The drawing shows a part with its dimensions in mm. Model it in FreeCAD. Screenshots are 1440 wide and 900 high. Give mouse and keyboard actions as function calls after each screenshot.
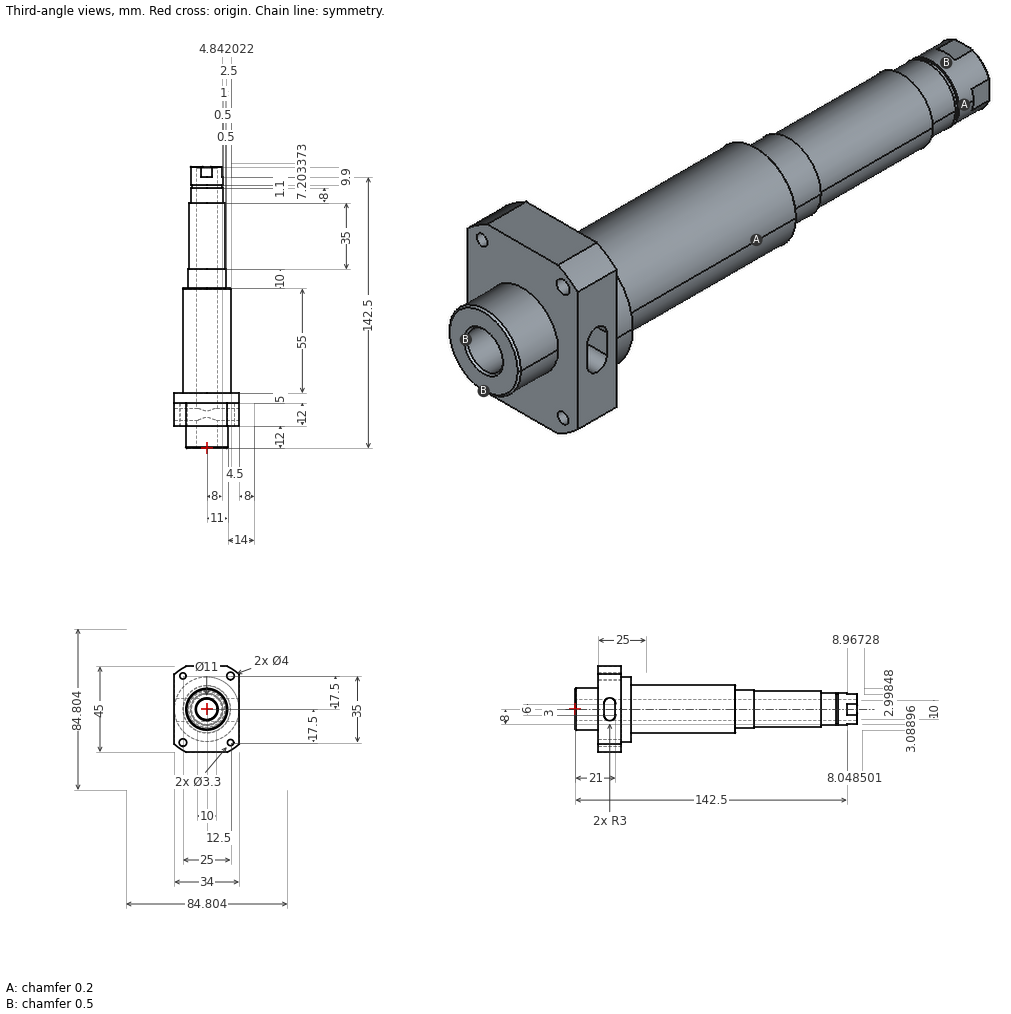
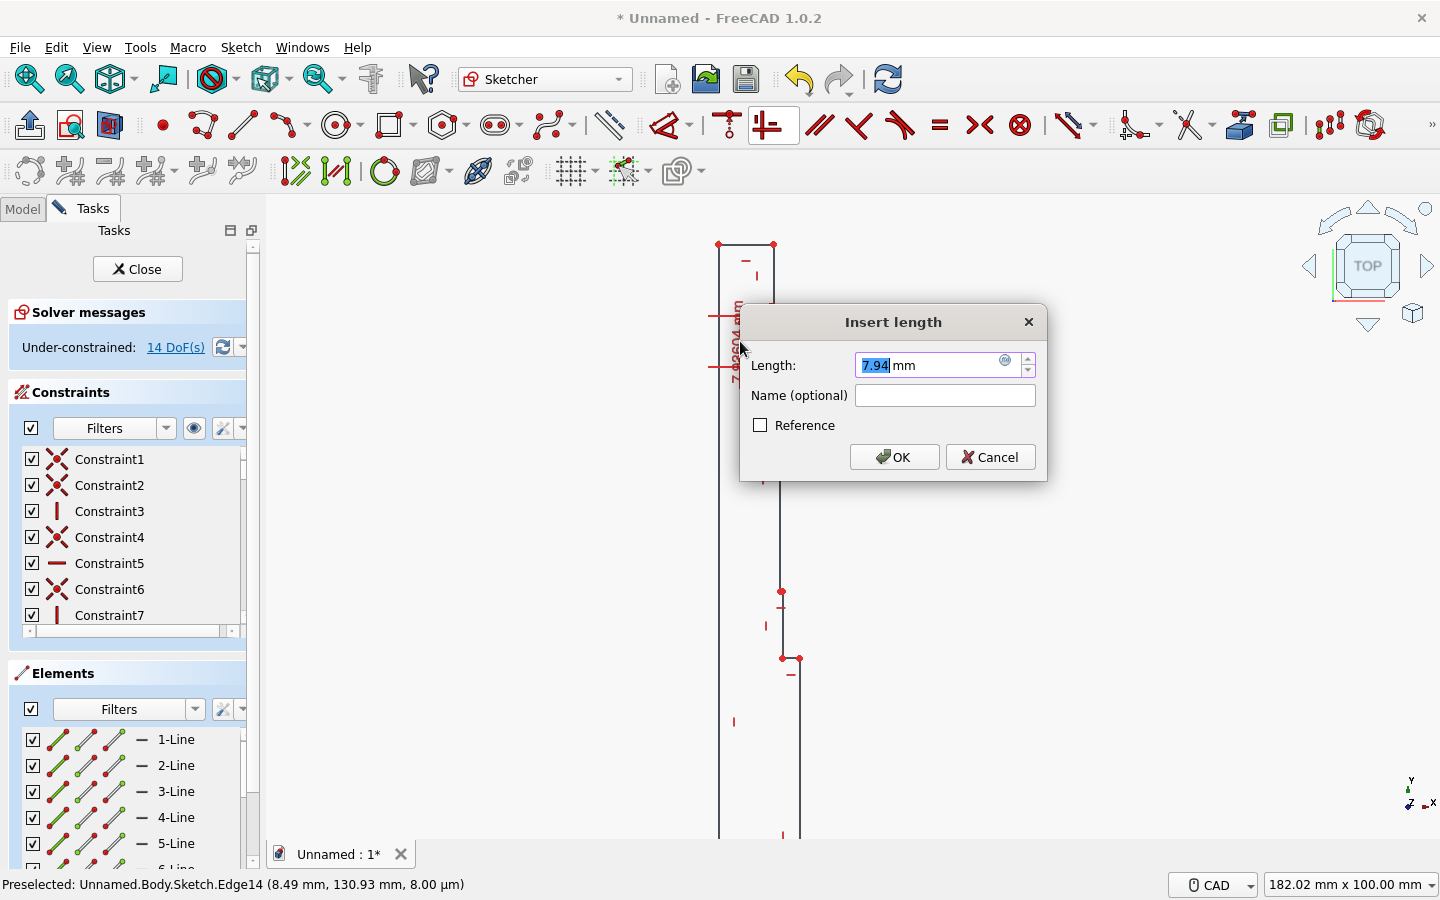
text(8)
key(Return)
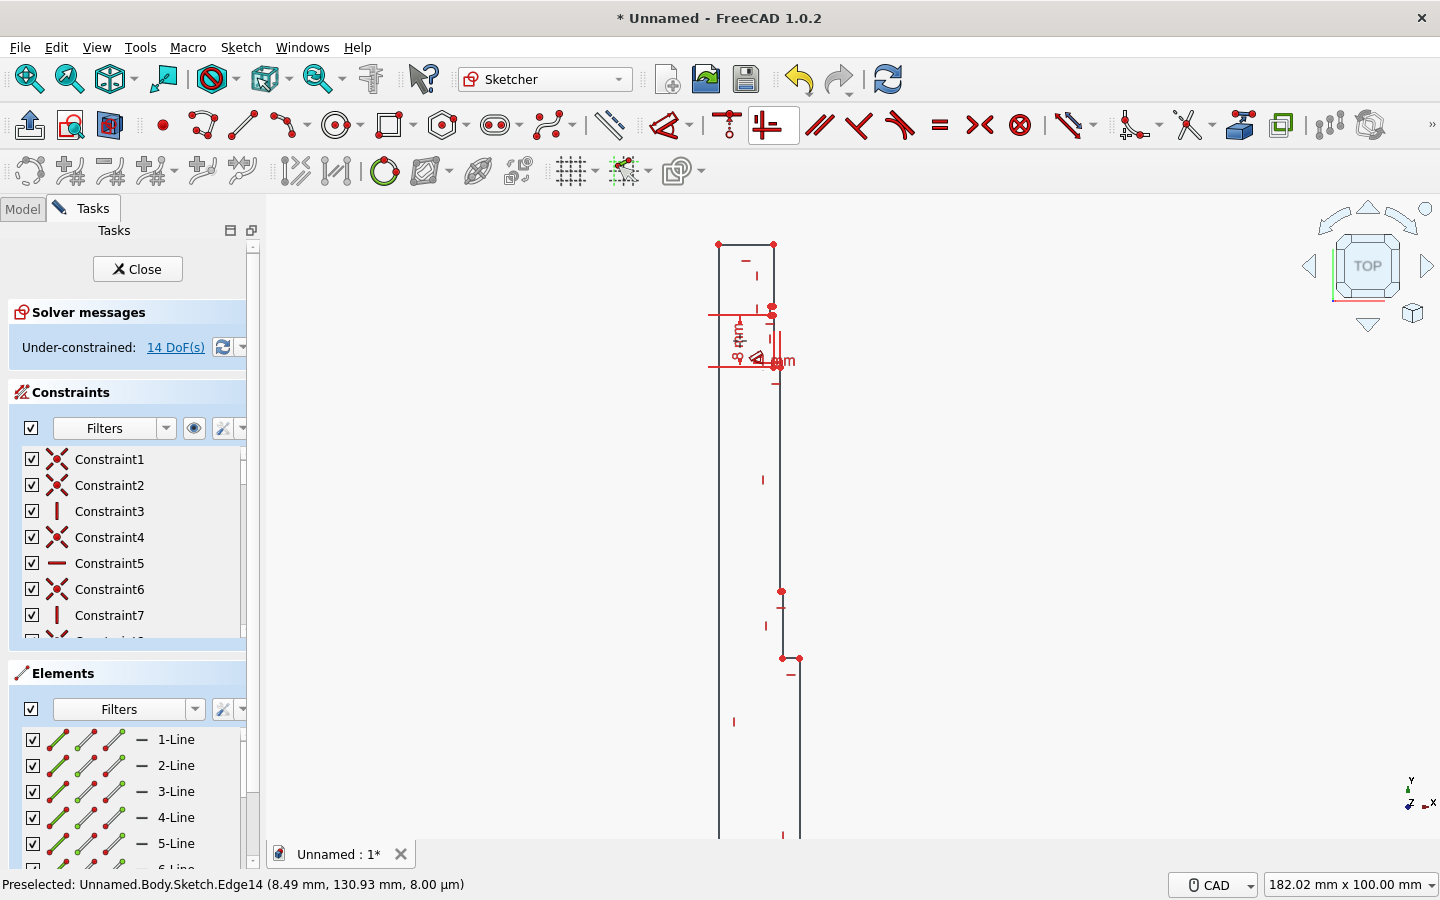
scroll(772, 350, down, 4)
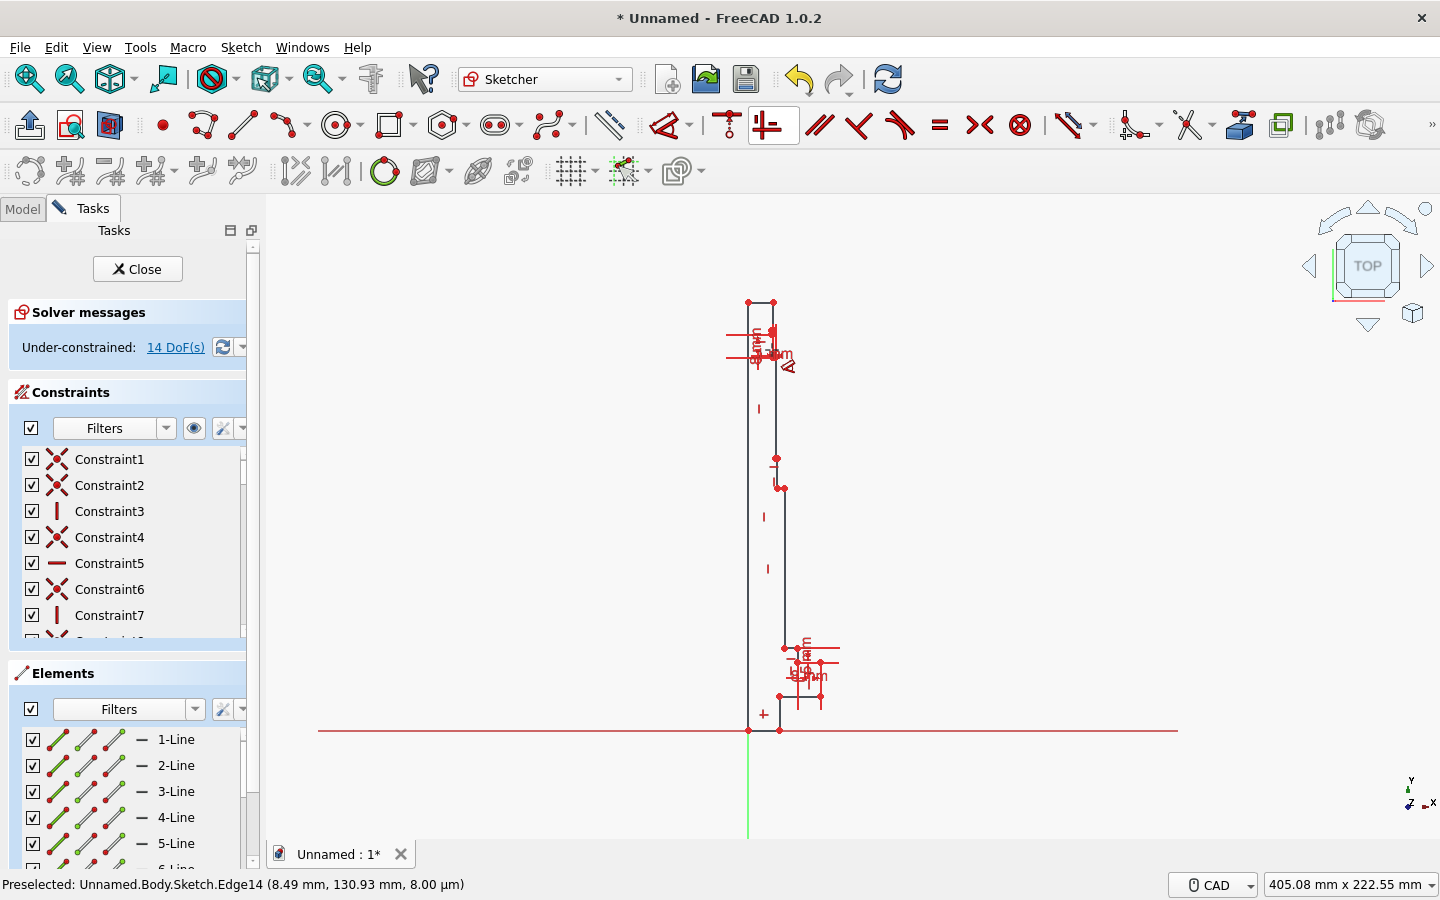
scroll(758, 731, up, 2)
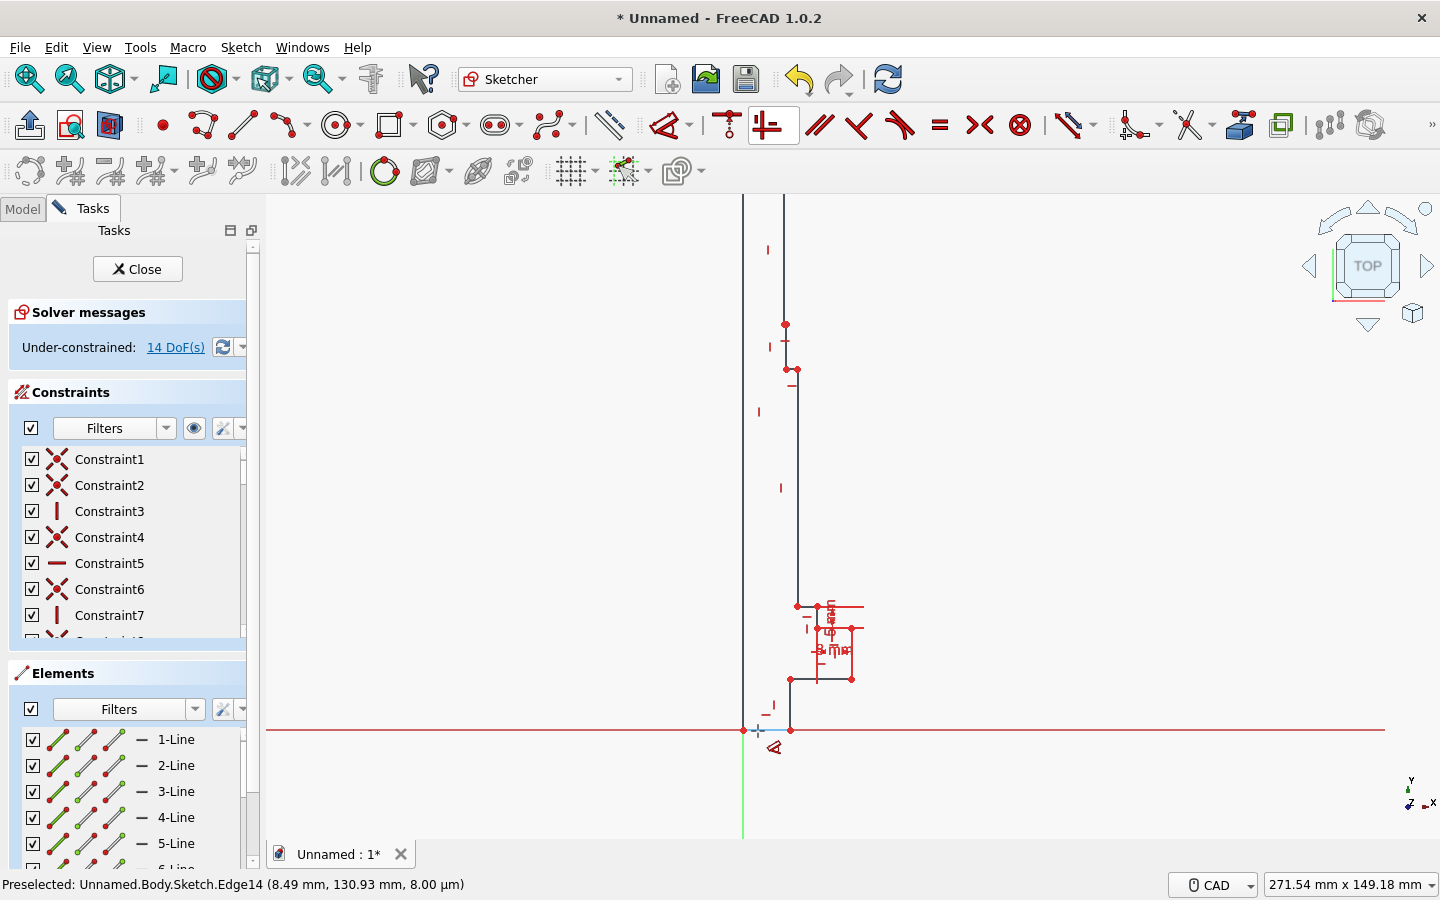
click(757, 730)
click(767, 764)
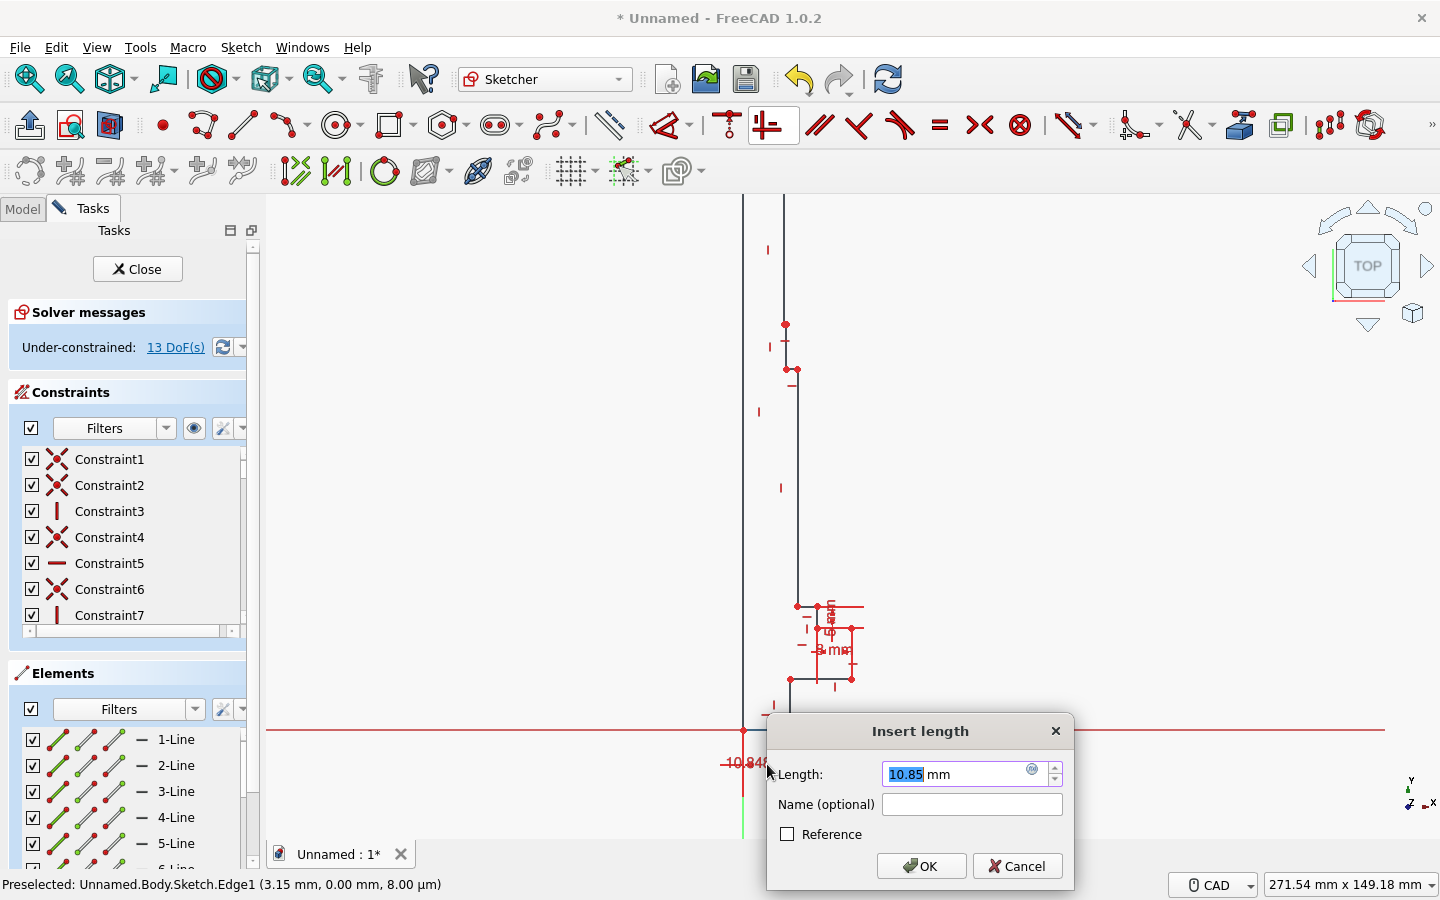
text(11)
key(Return)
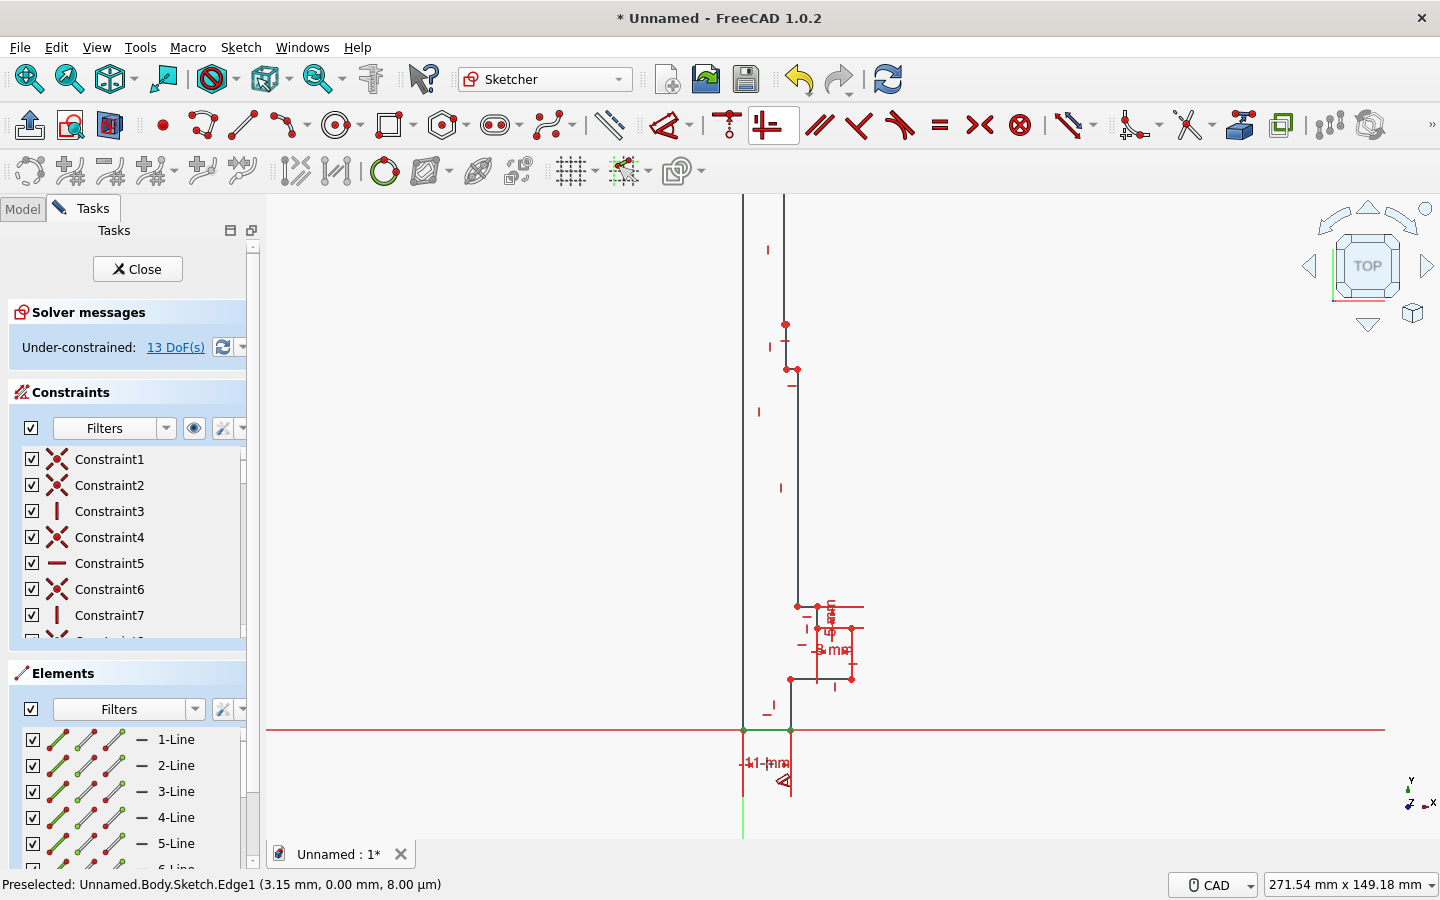
click(791, 715)
click(757, 705)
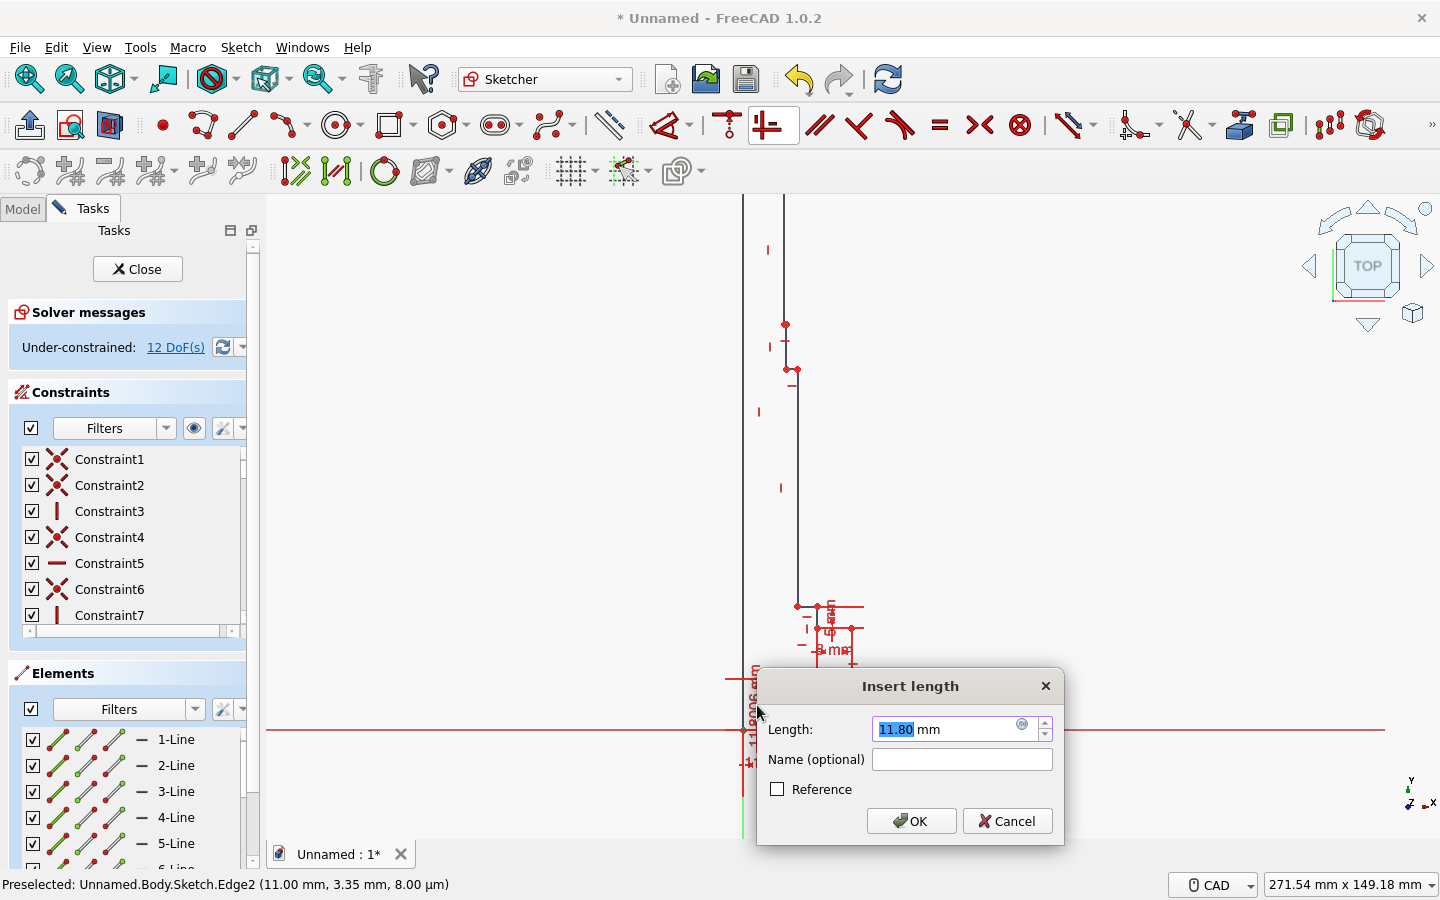
text(12)
key(Return)